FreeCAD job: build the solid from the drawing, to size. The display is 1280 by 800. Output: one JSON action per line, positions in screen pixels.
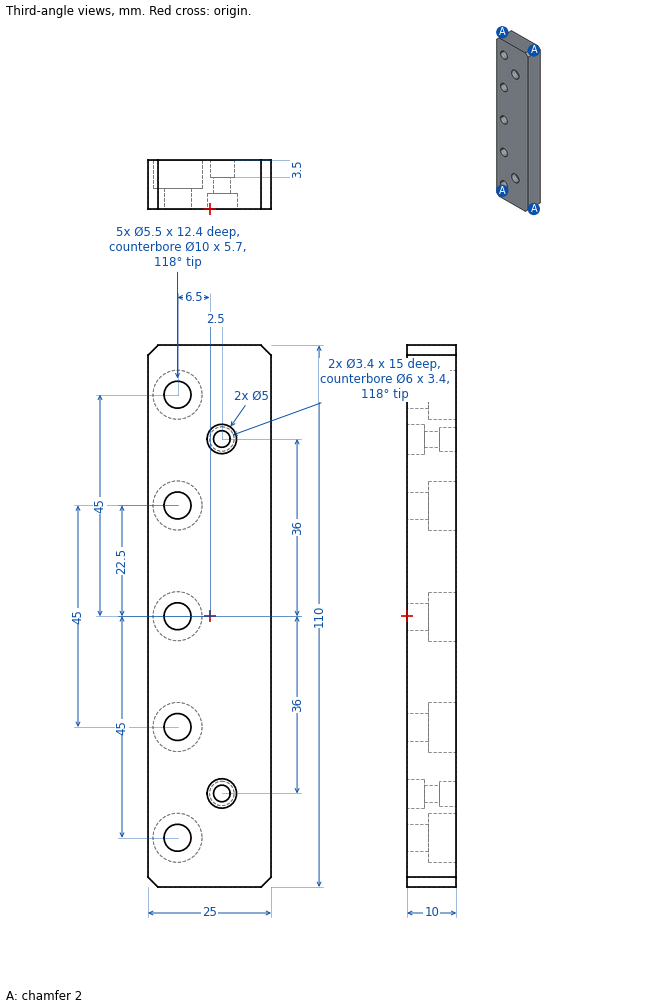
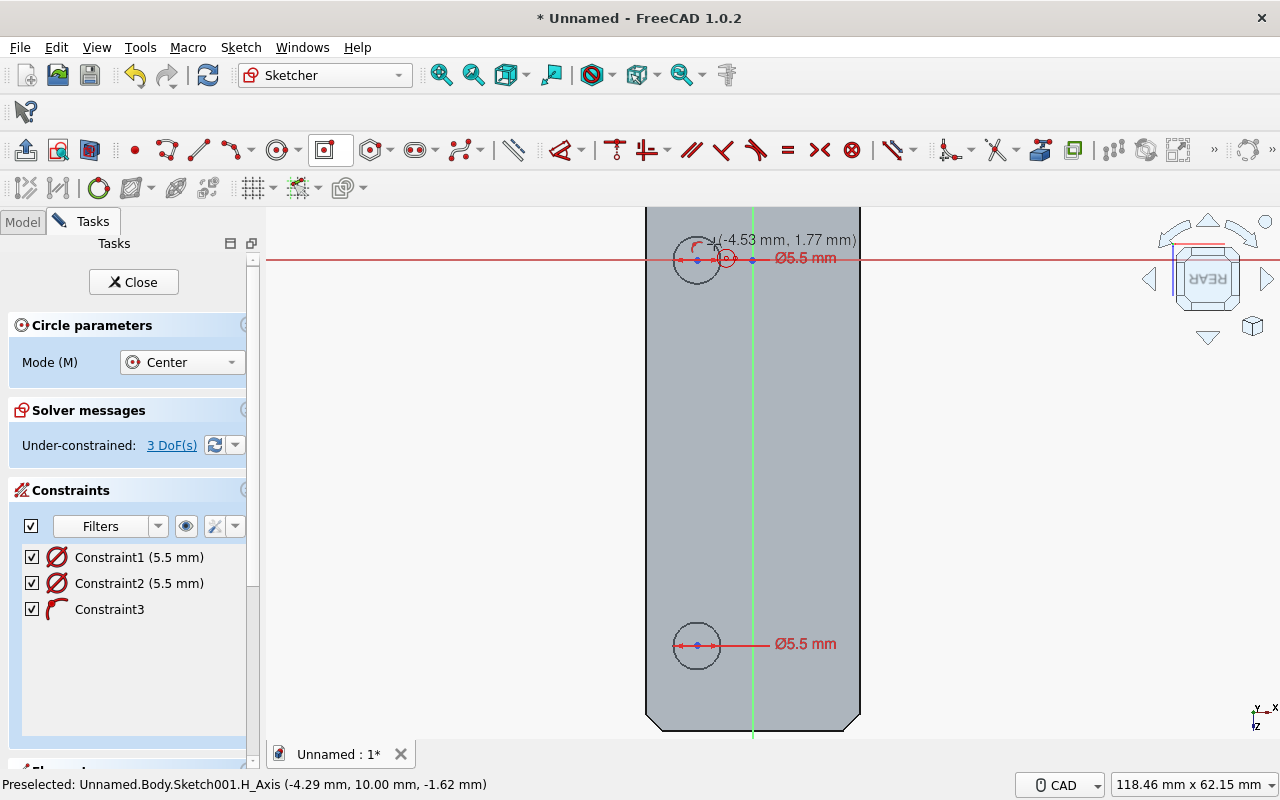
{"action": "scroll", "coordinate": [697, 647], "scroll_direction": "down", "scroll_amount": 4}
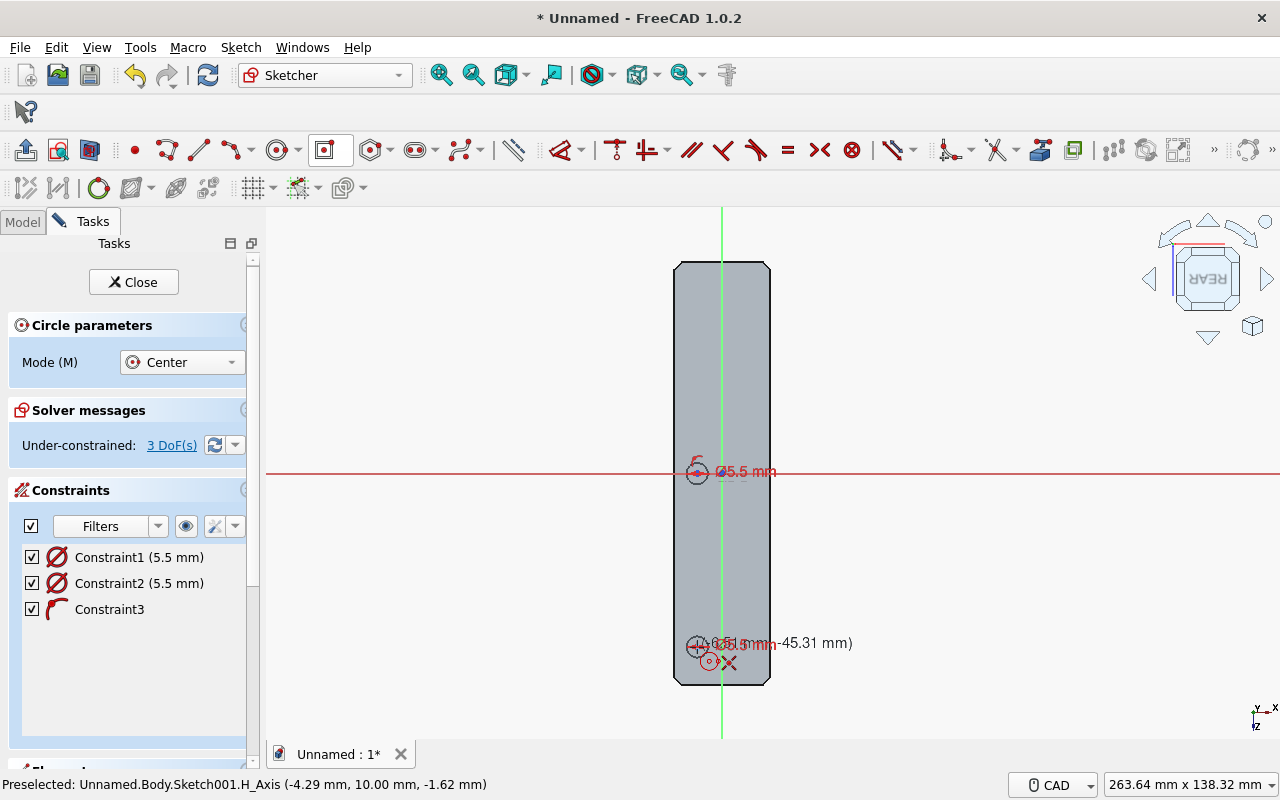
{"action": "scroll", "coordinate": [697, 301], "scroll_direction": "up", "scroll_amount": 4}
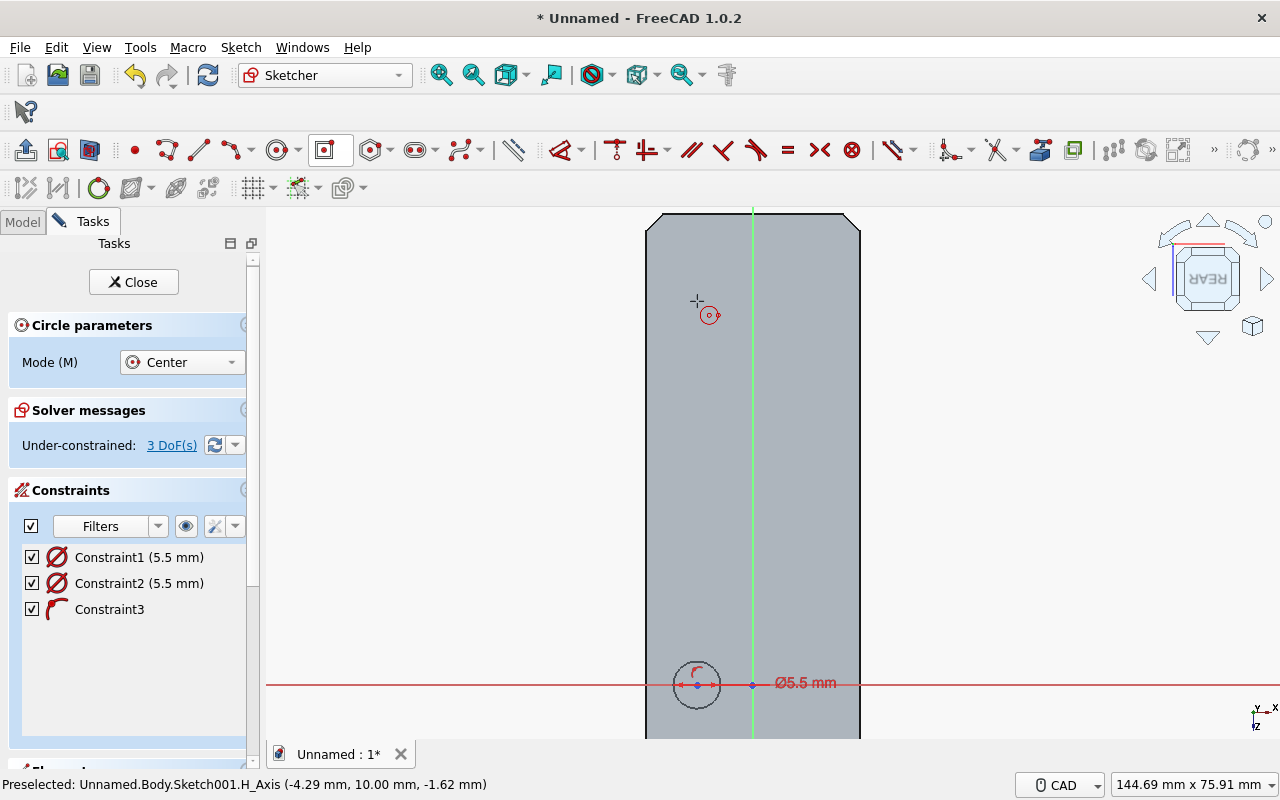
{"action": "left_click", "coordinate": [697, 300]}
{"action": "mouse_move", "coordinate": [714, 283]}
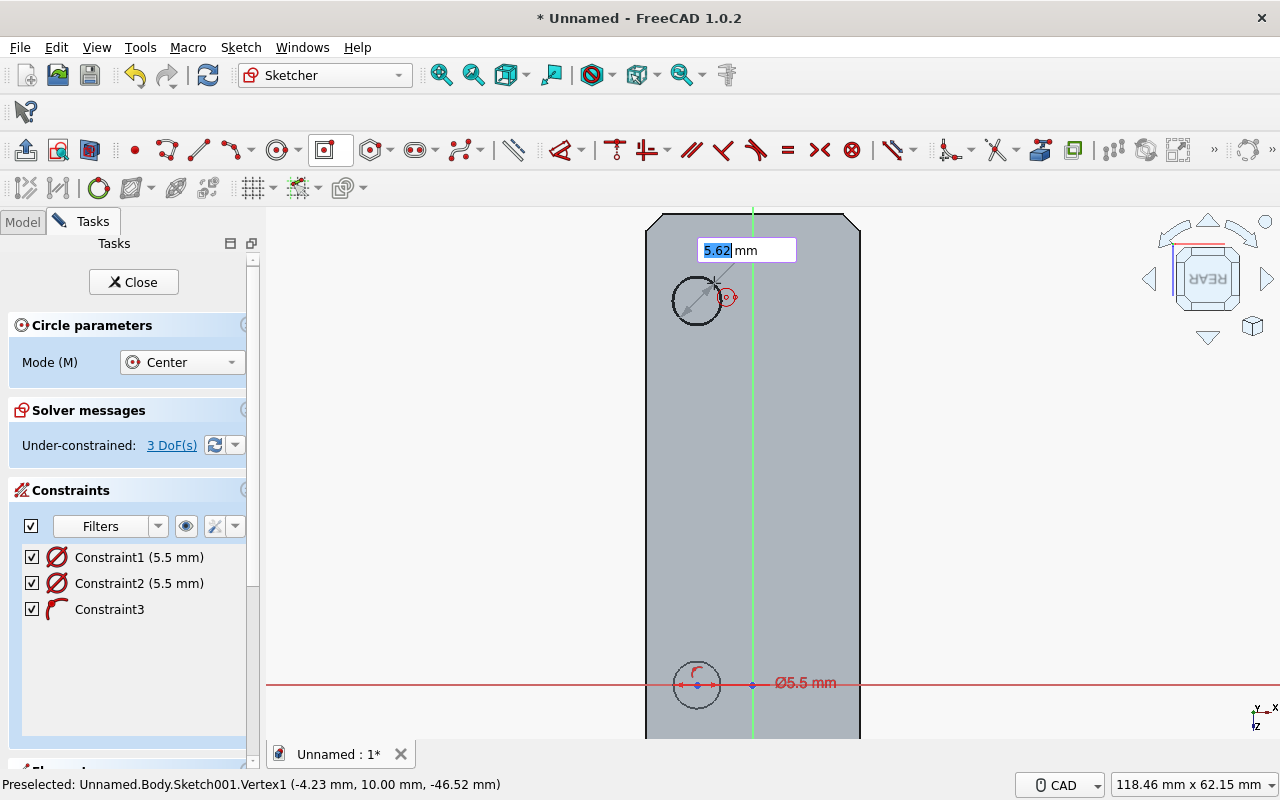
{"action": "type", "text": "5.5"}
{"action": "key", "text": "Return"}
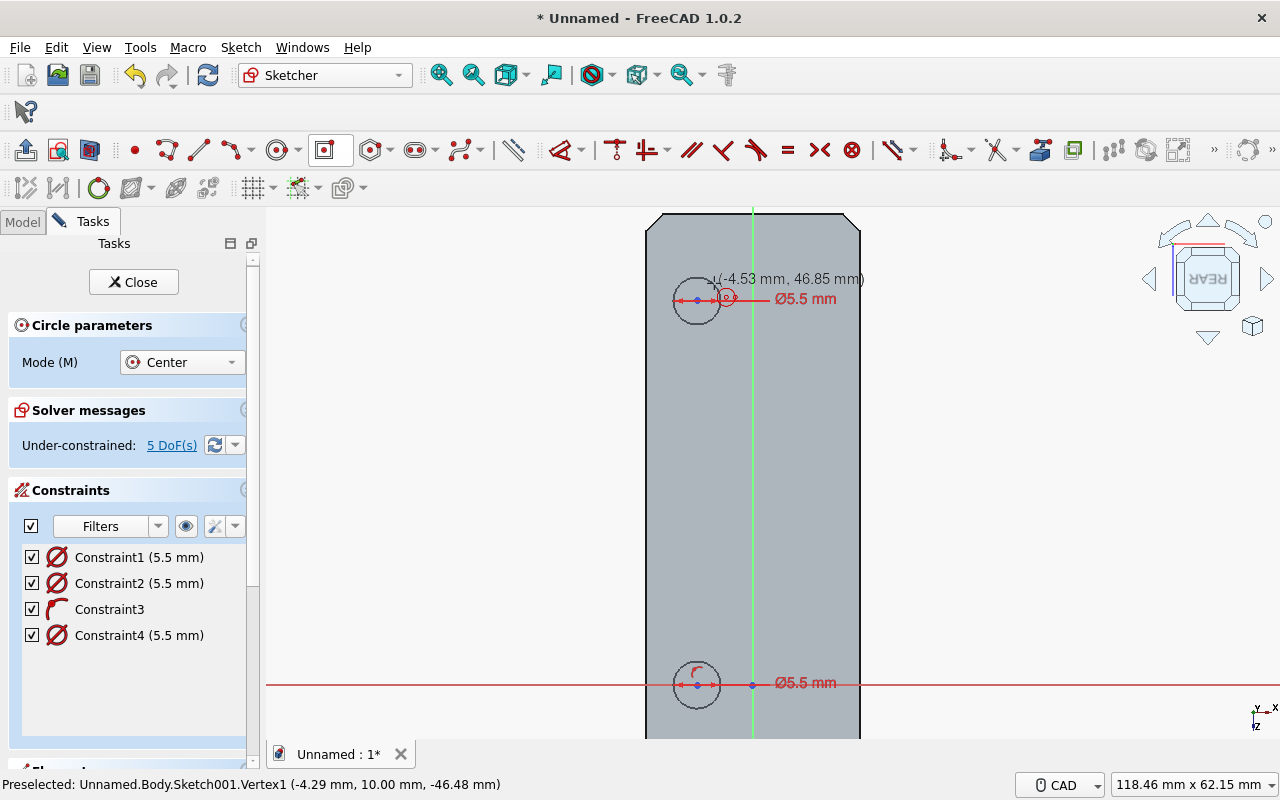
{"action": "scroll", "coordinate": [697, 300], "scroll_direction": "down", "scroll_amount": 4}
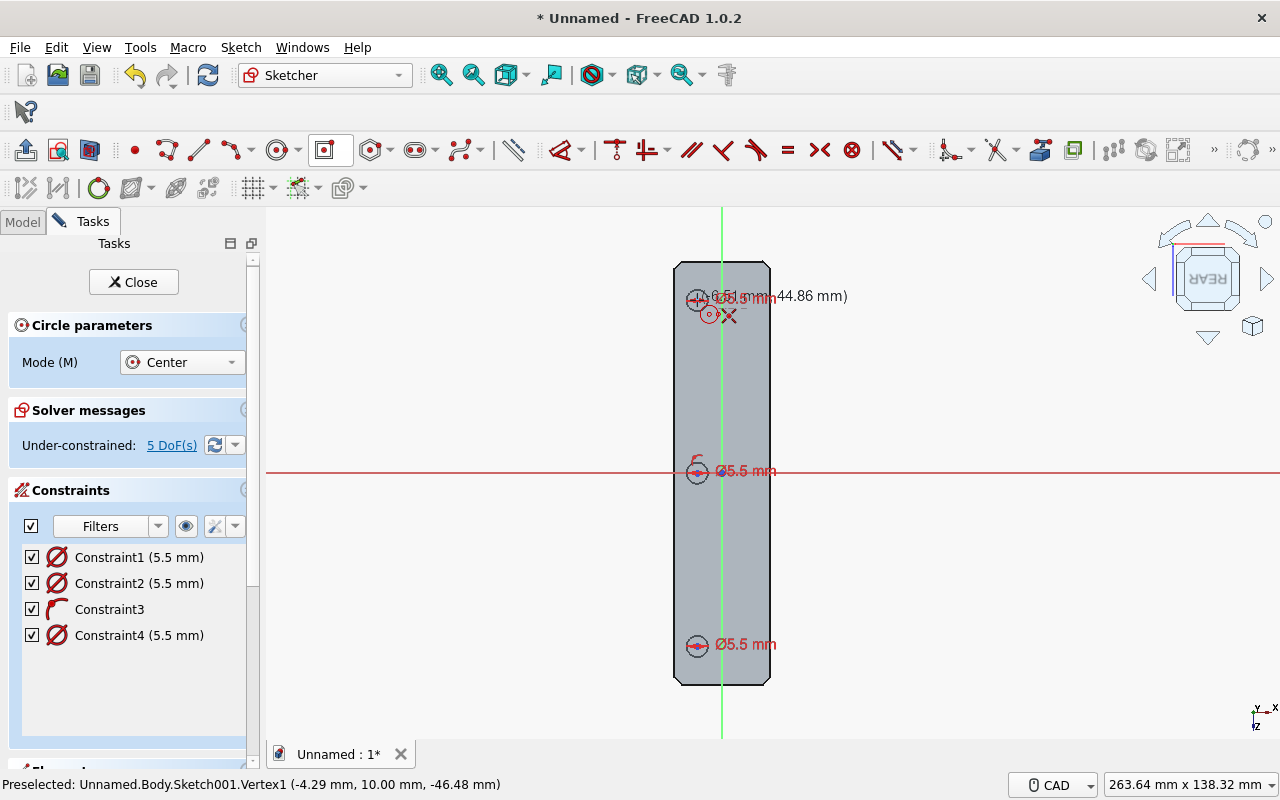
{"action": "scroll", "coordinate": [697, 560], "scroll_direction": "up", "scroll_amount": 4}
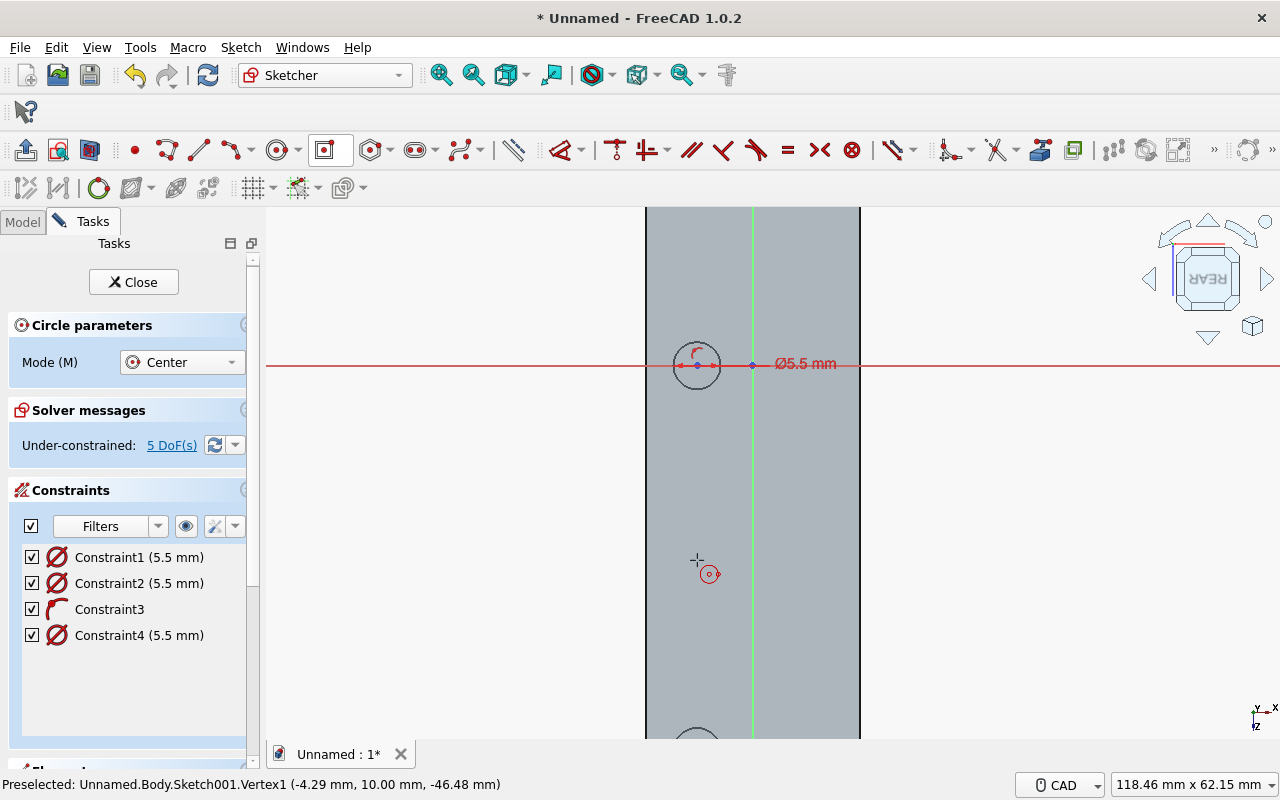
{"action": "left_click", "coordinate": [697, 558]}
{"action": "mouse_move", "coordinate": [714, 542]}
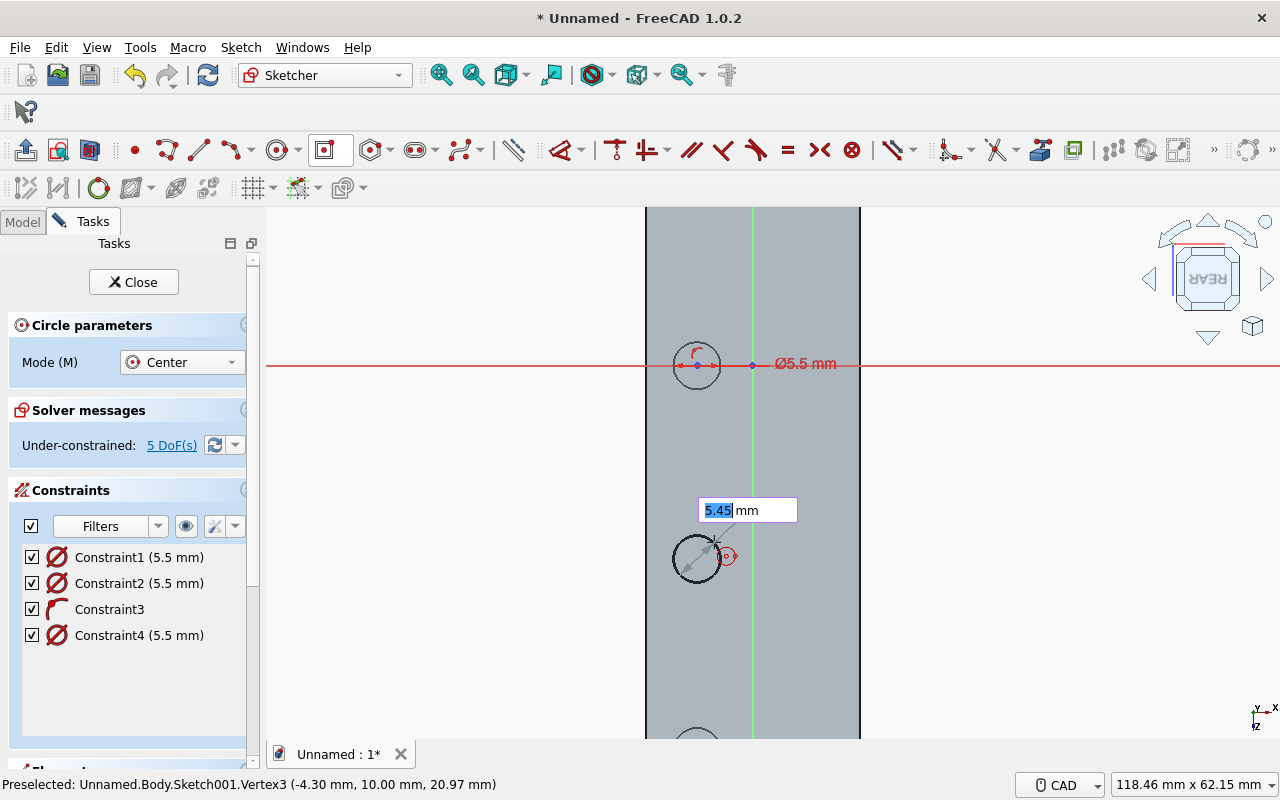
{"action": "type", "text": "5.5"}
{"action": "key", "text": "Return"}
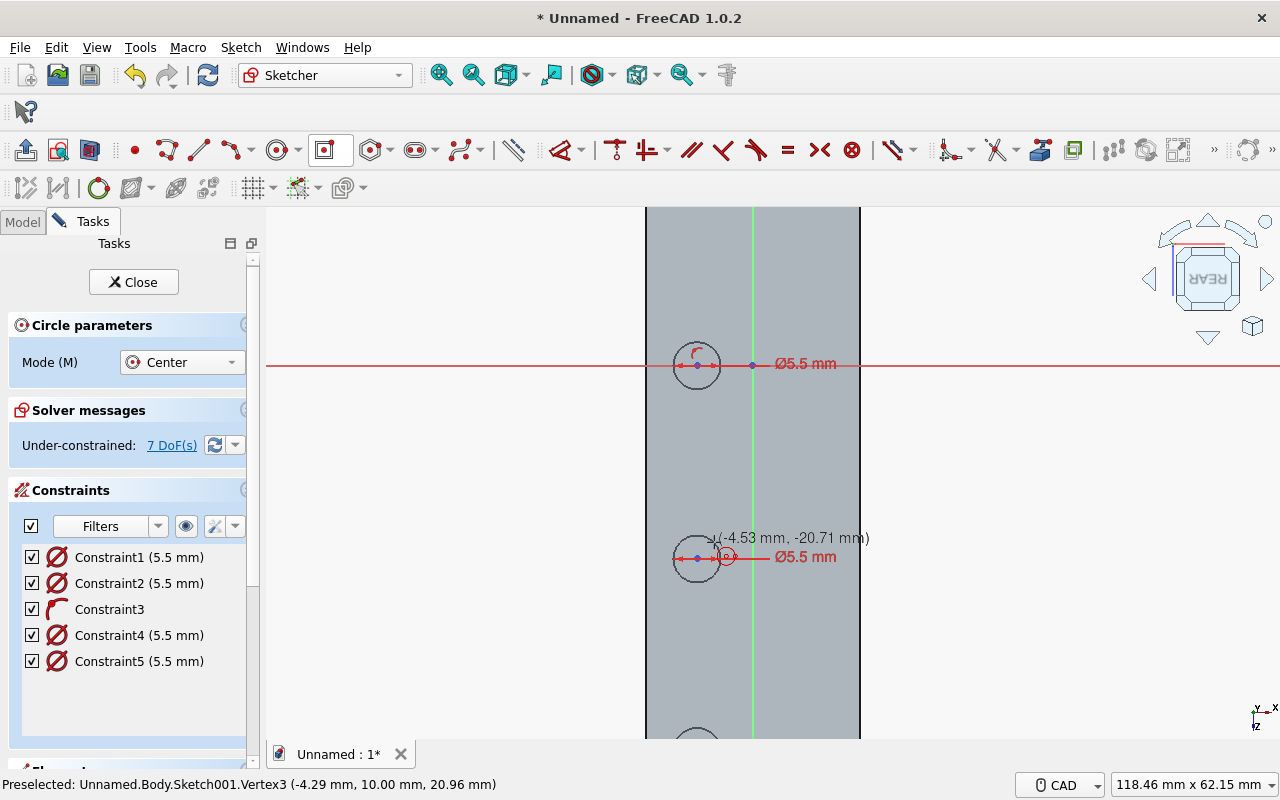
{"action": "scroll", "coordinate": [697, 560], "scroll_direction": "down", "scroll_amount": 4}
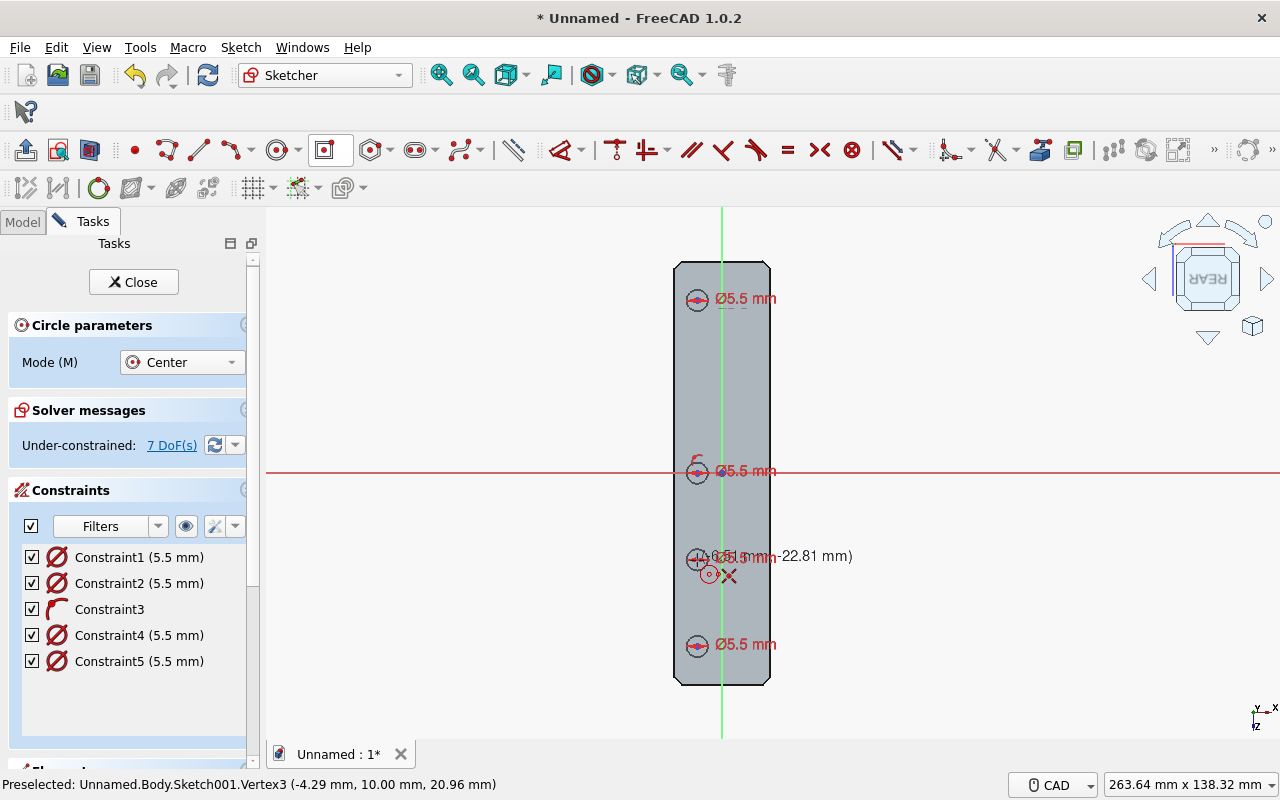
{"action": "scroll", "coordinate": [697, 387], "scroll_direction": "up", "scroll_amount": 4}